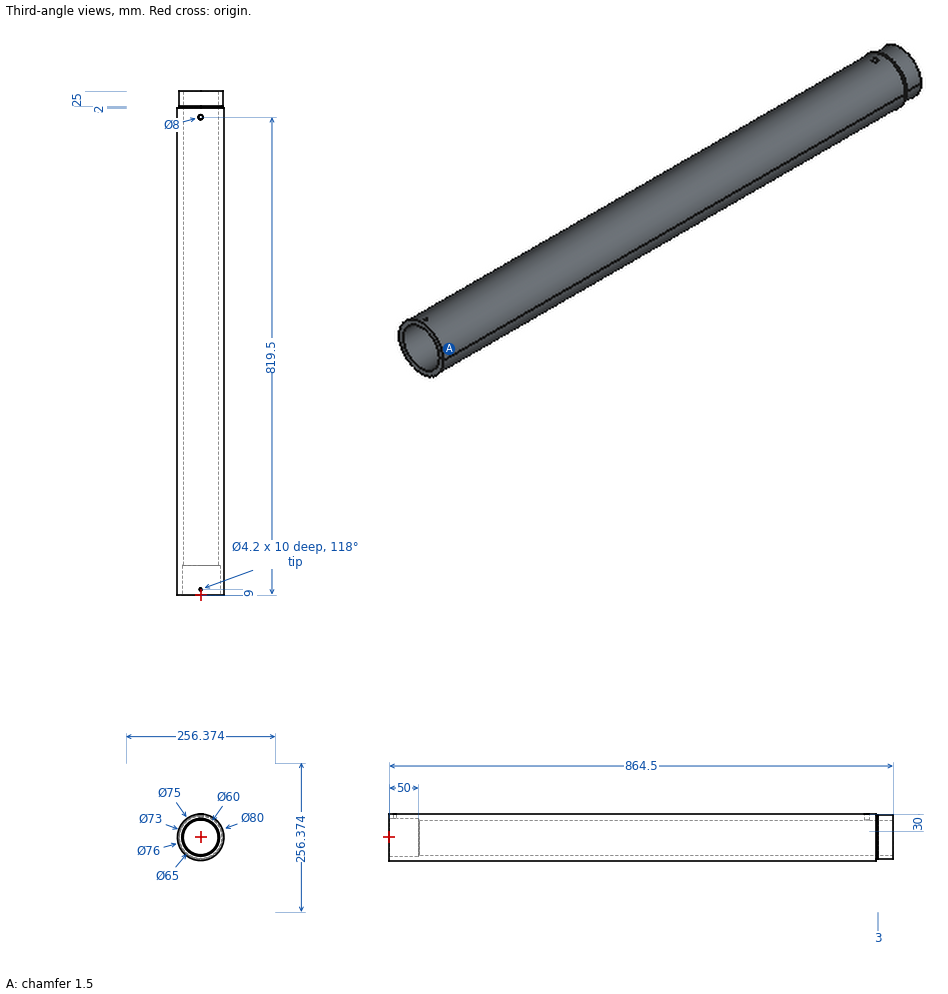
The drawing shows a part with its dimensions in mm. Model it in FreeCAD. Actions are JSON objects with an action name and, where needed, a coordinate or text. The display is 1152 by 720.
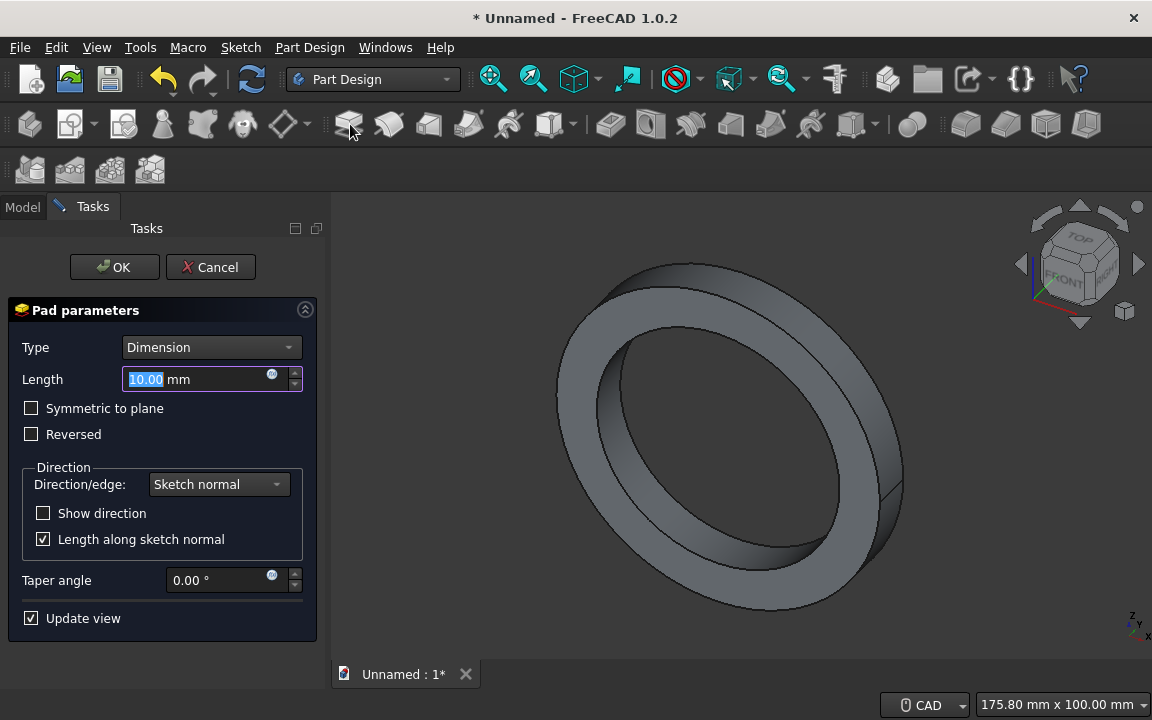
{"action": "type", "text": "864.5"}
{"action": "key", "text": "Tab"}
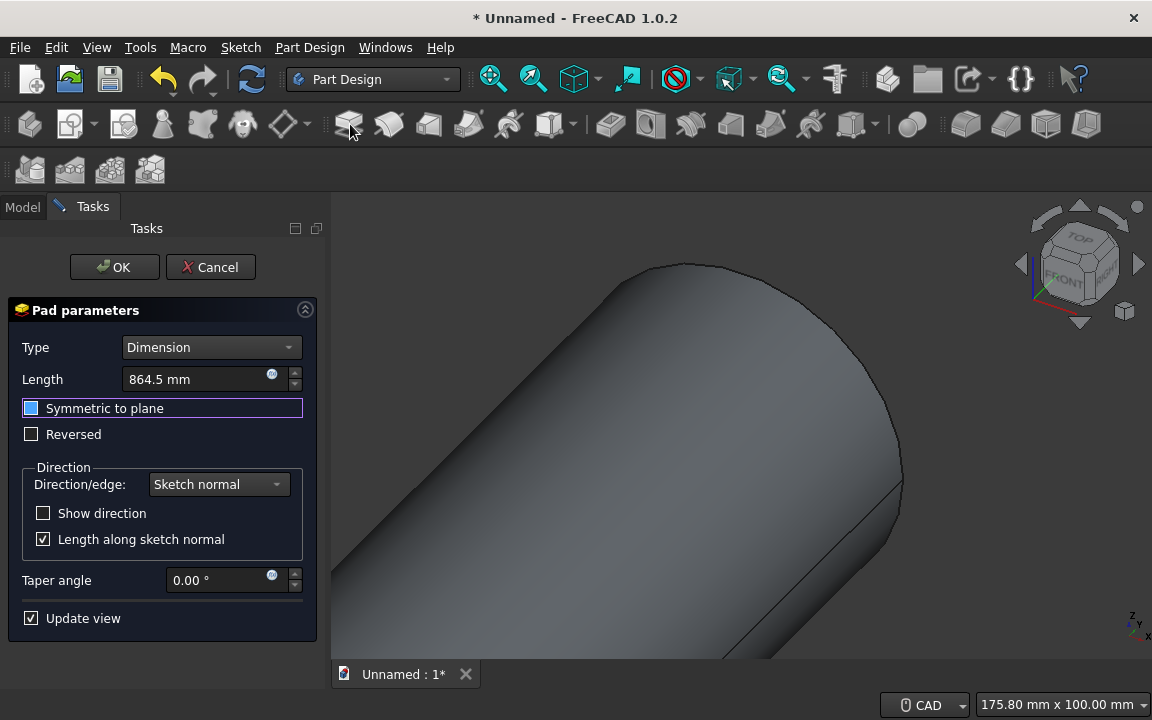
{"action": "left_click", "coordinate": [30, 434]}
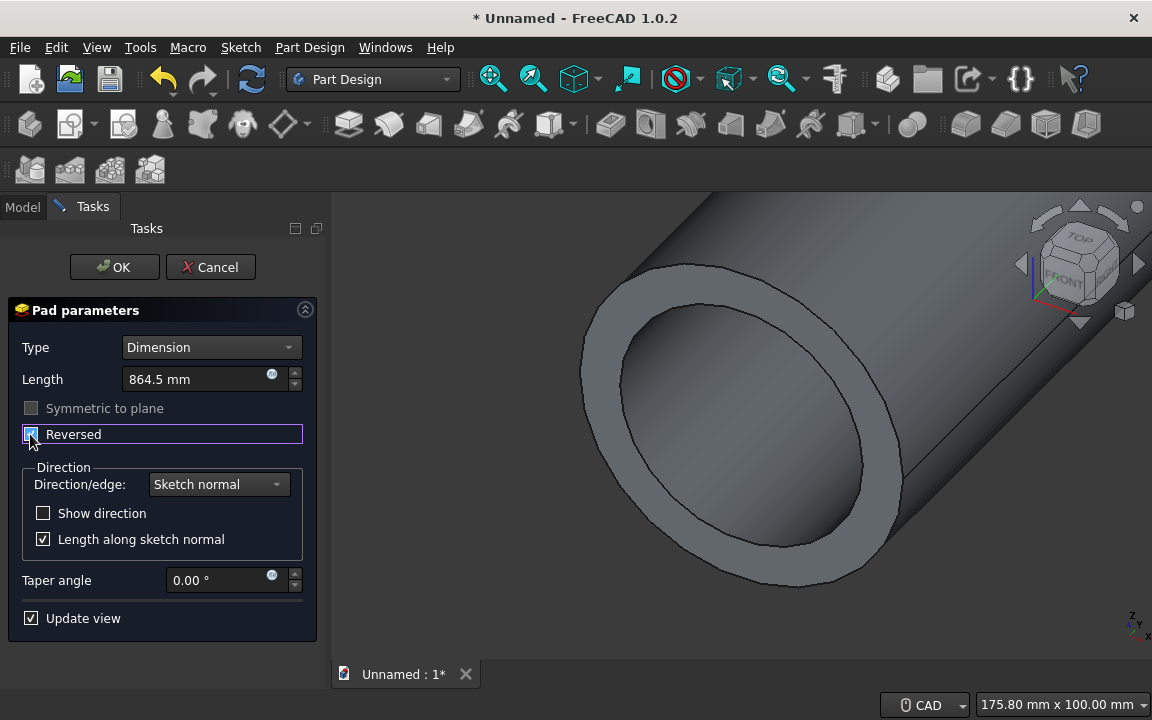
{"action": "left_click", "coordinate": [115, 267]}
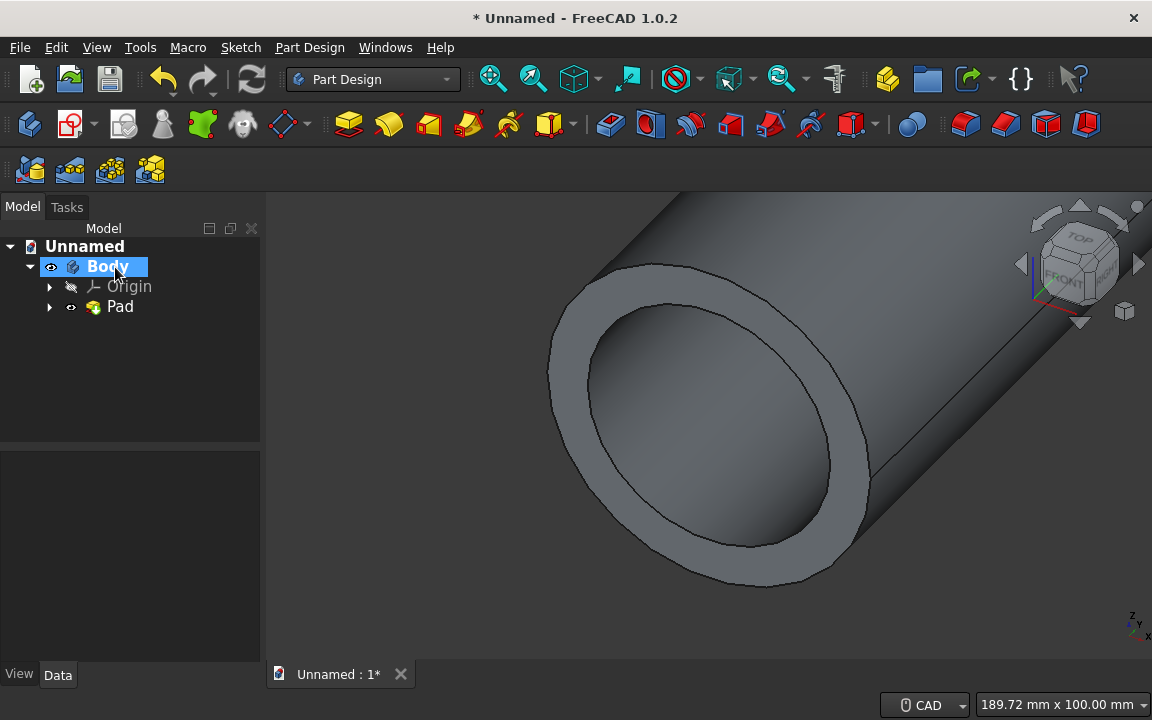
{"action": "key", "text": "v f"}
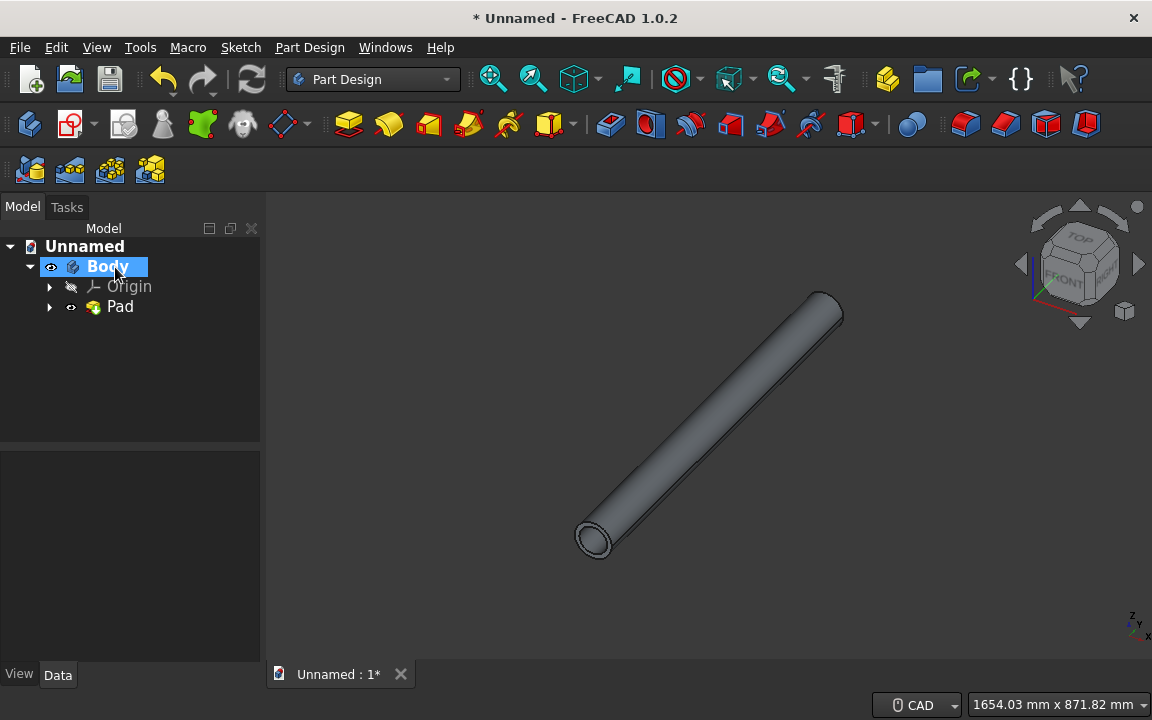
{"action": "key", "text": "4"}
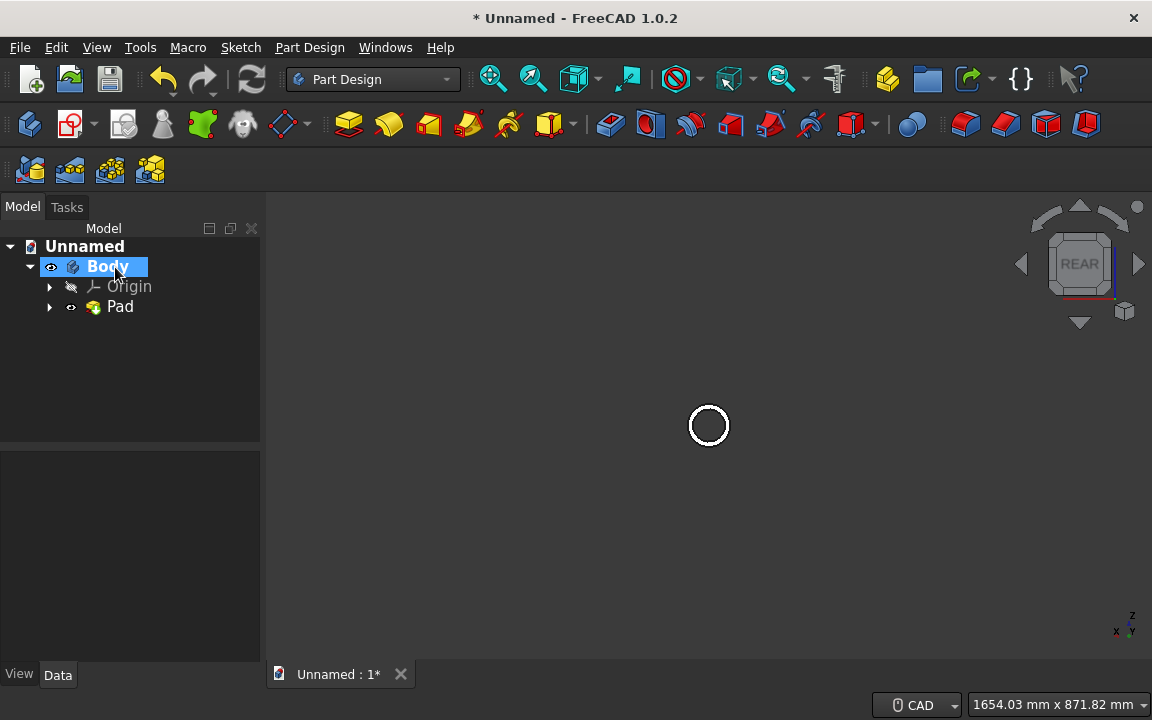
{"action": "left_click", "coordinate": [494, 80]}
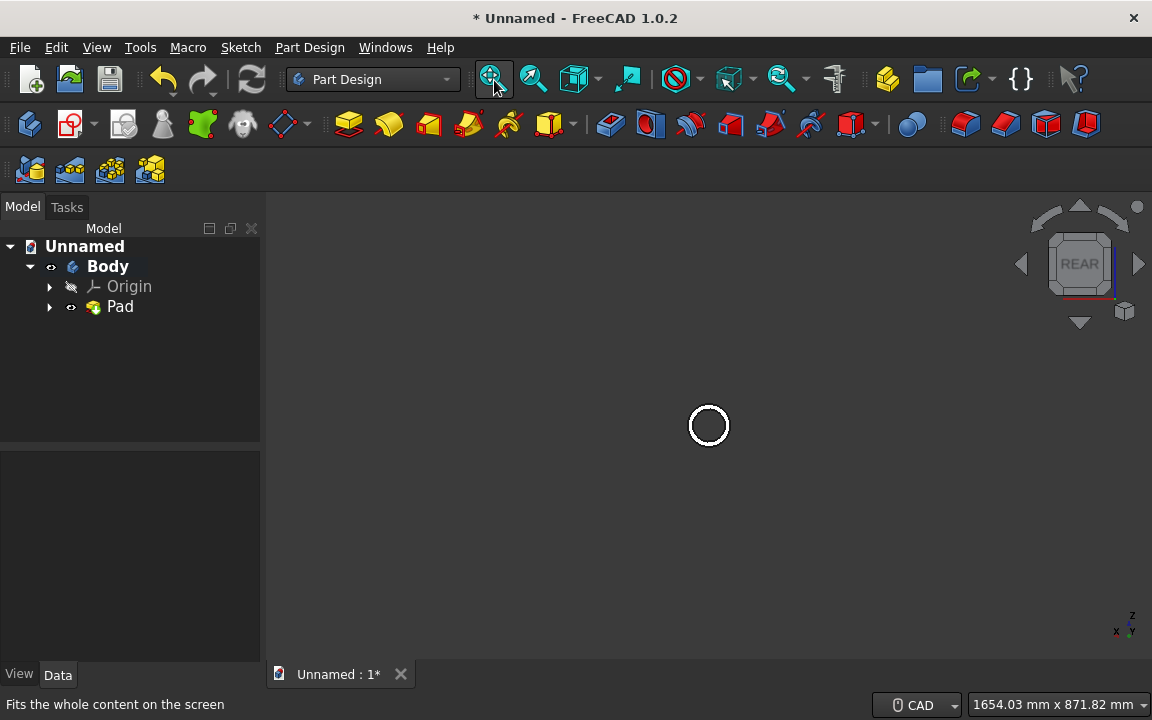
{"action": "scroll", "coordinate": [691, 425], "scroll_direction": "up", "scroll_amount": 9}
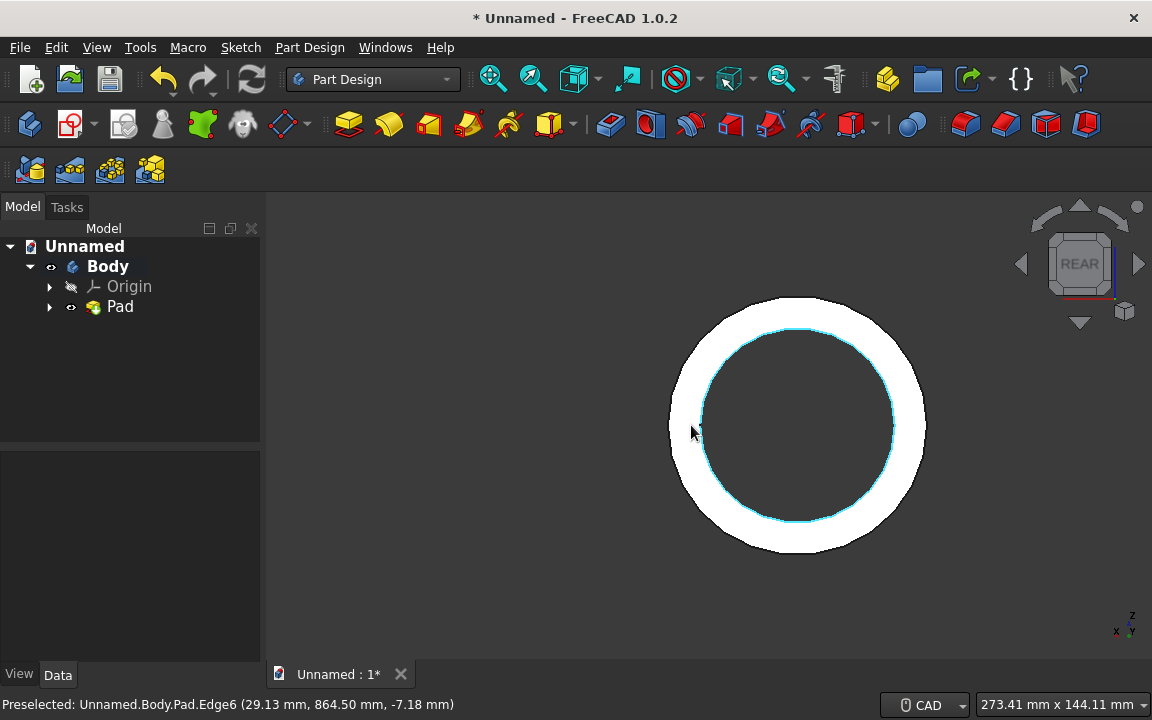
{"action": "left_click", "coordinate": [686, 425]}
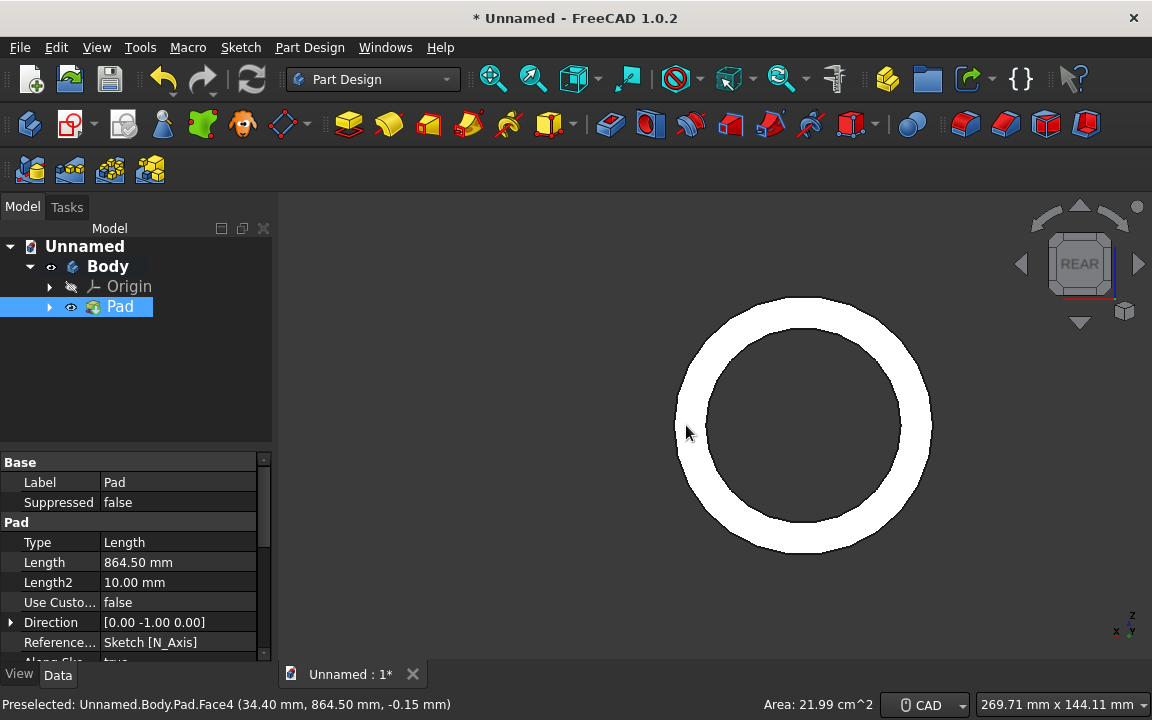
{"action": "left_click", "coordinate": [70, 124]}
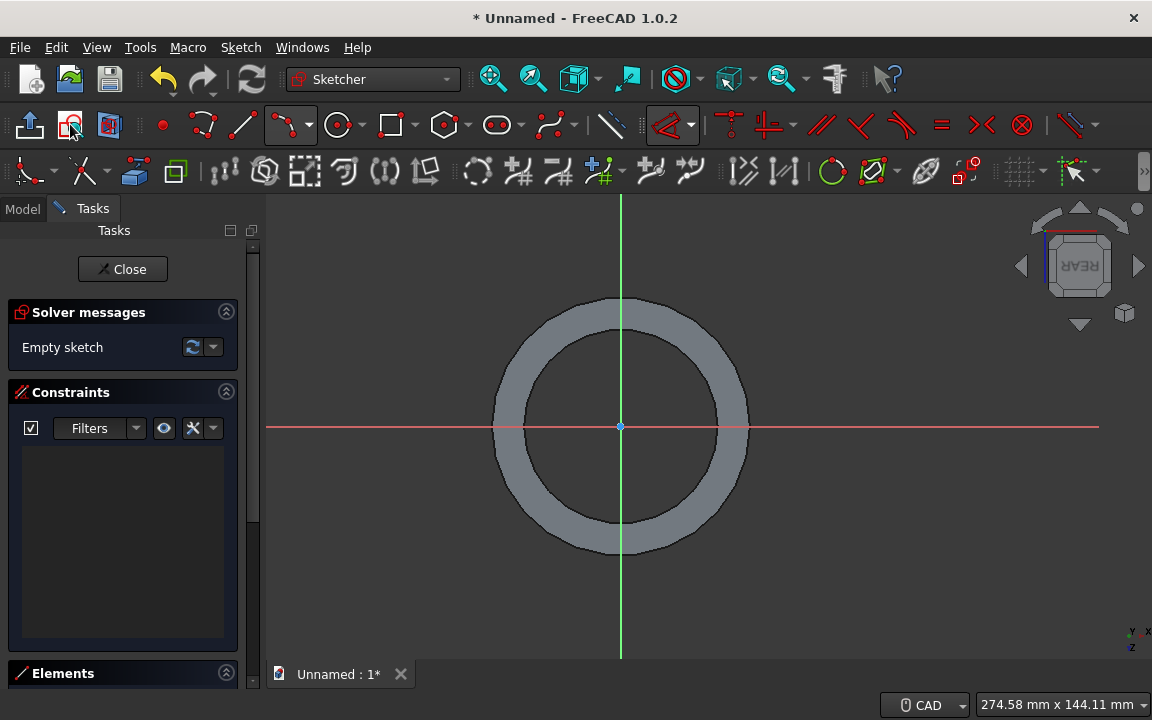
{"action": "scroll", "coordinate": [652, 427], "scroll_direction": "down", "scroll_amount": 5}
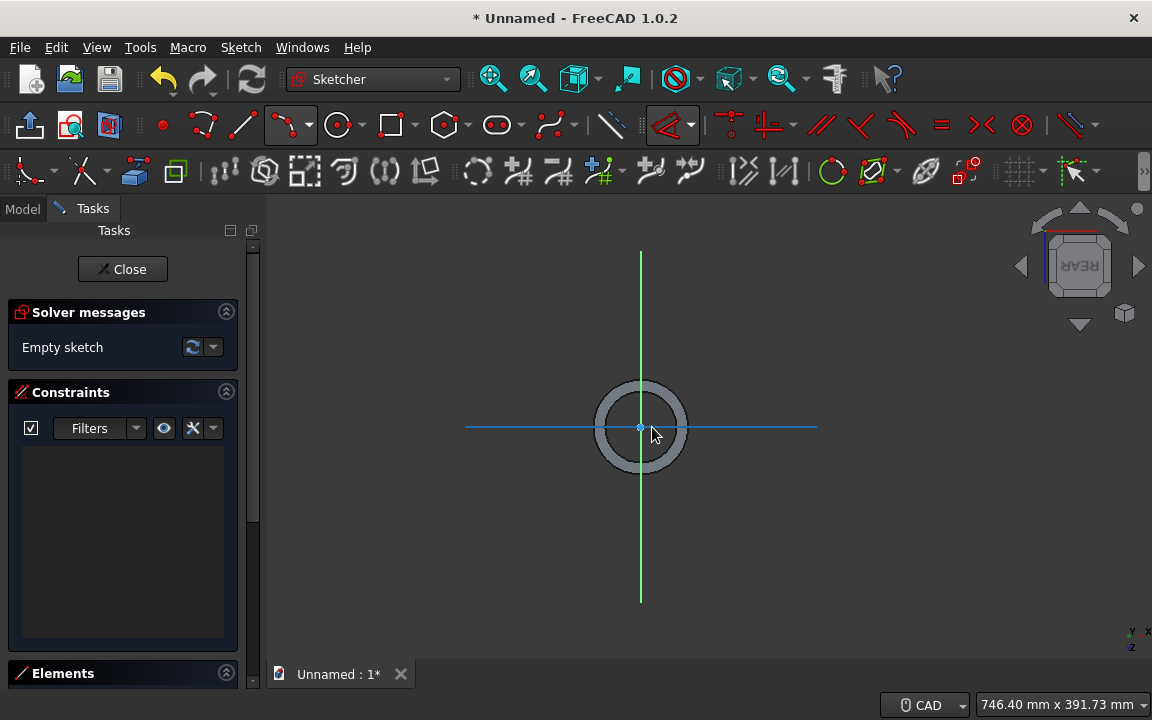
{"action": "left_click", "coordinate": [418, 126]}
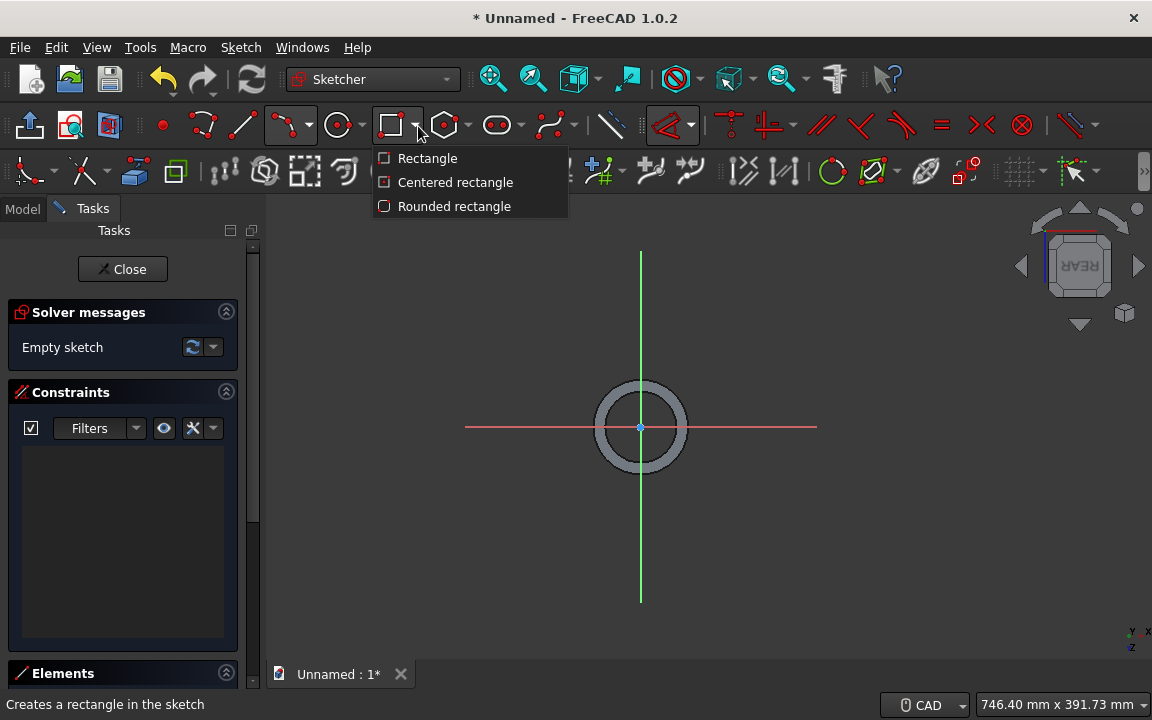
{"action": "left_click", "coordinate": [470, 182]}